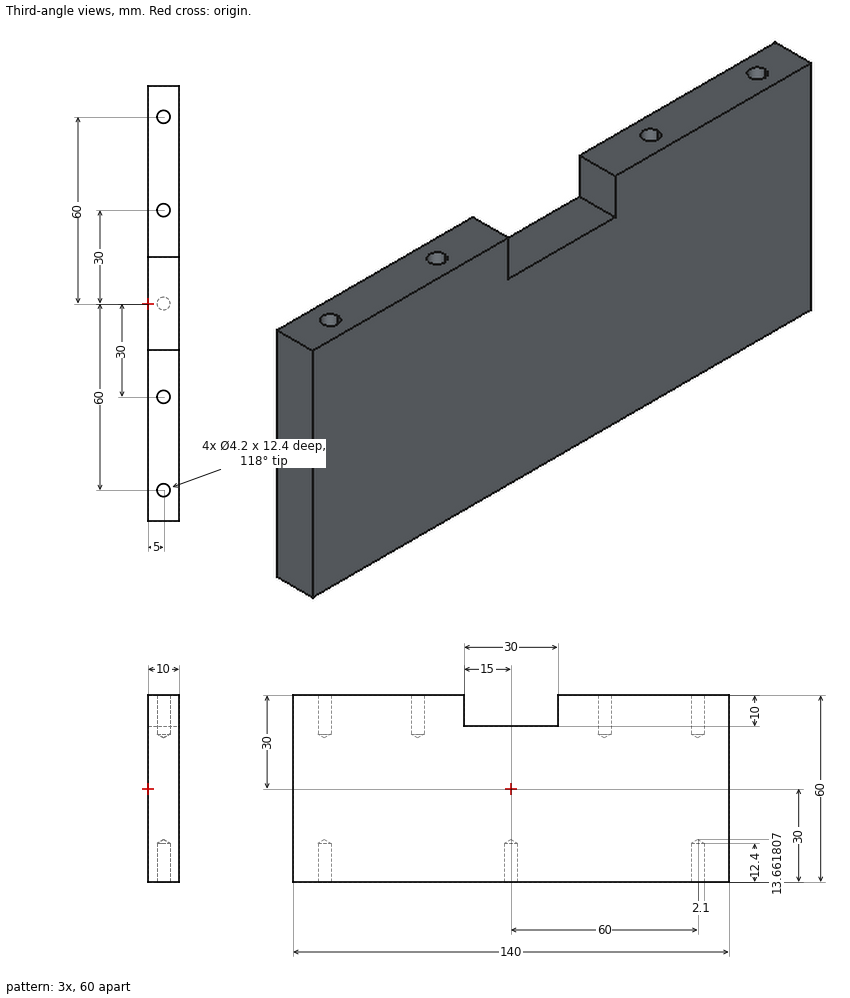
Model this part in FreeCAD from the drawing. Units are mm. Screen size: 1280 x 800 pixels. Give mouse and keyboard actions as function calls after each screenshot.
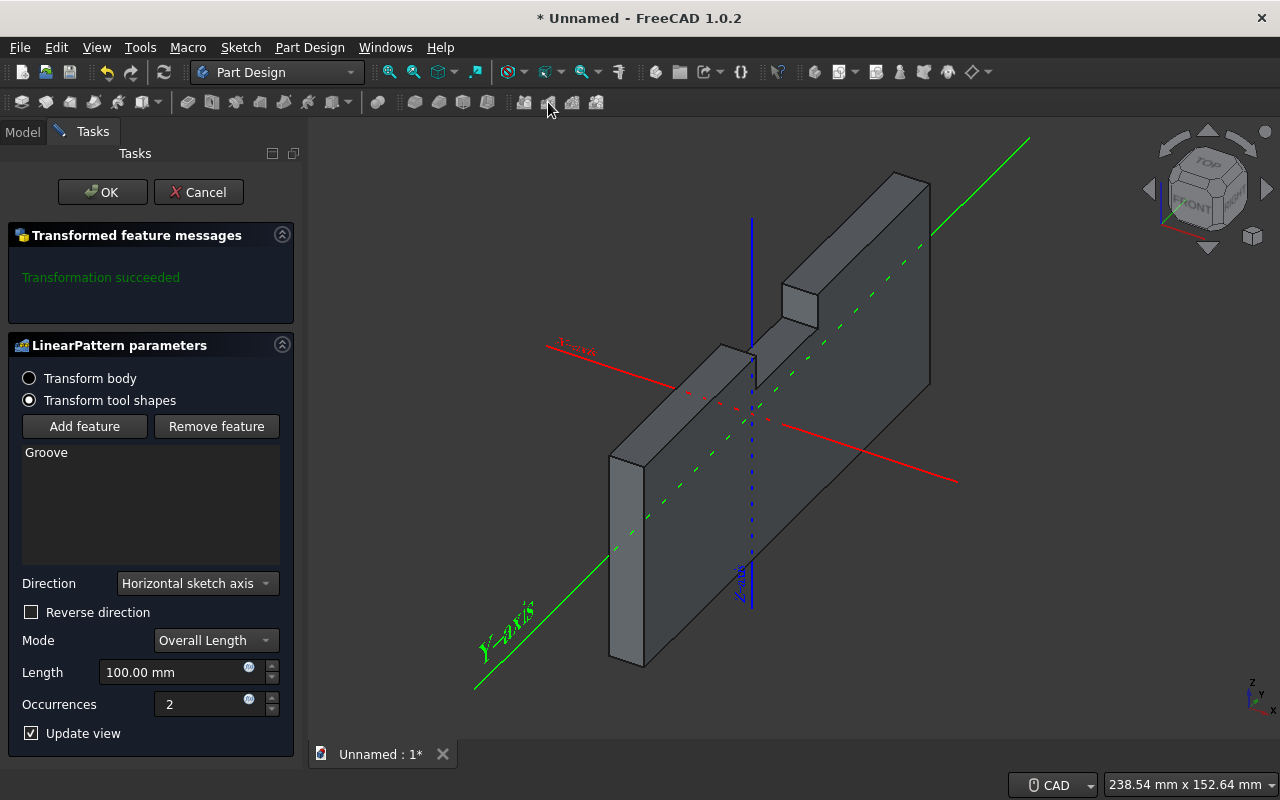
click(198, 584)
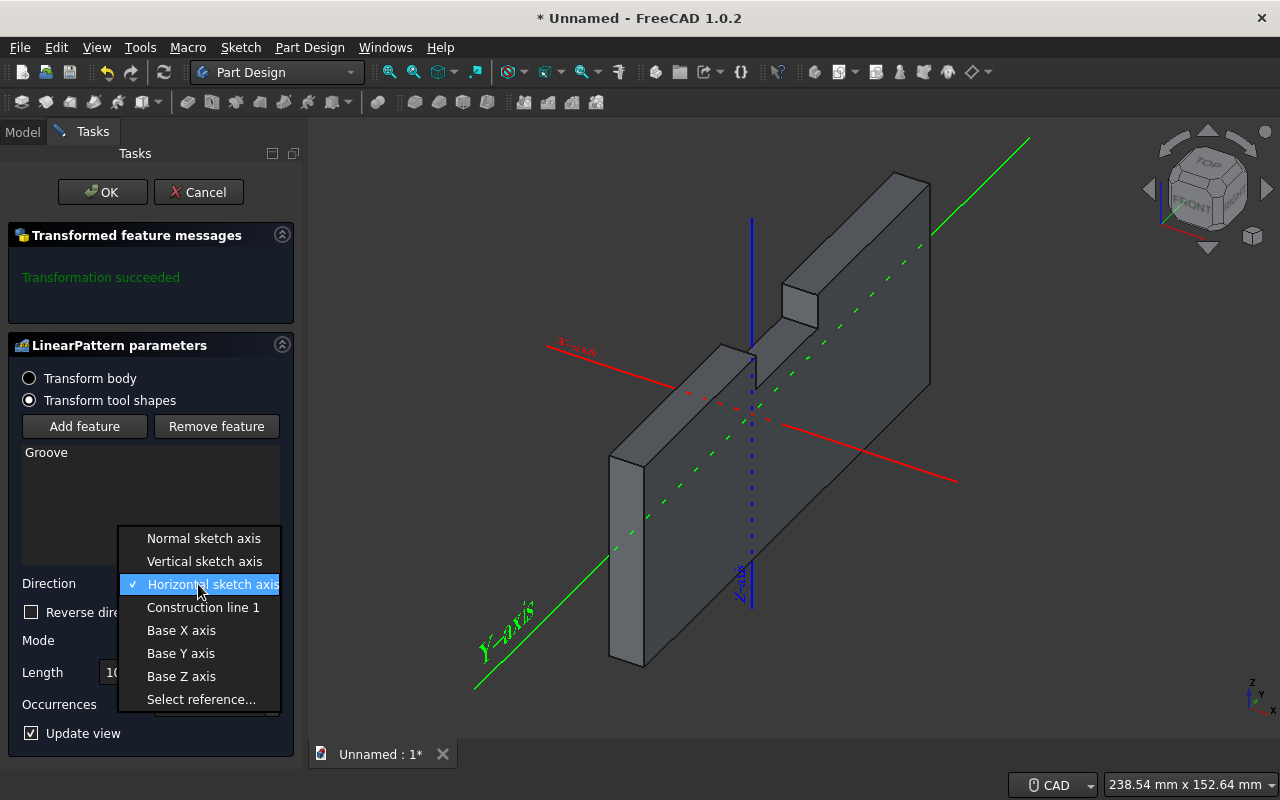
click(198, 654)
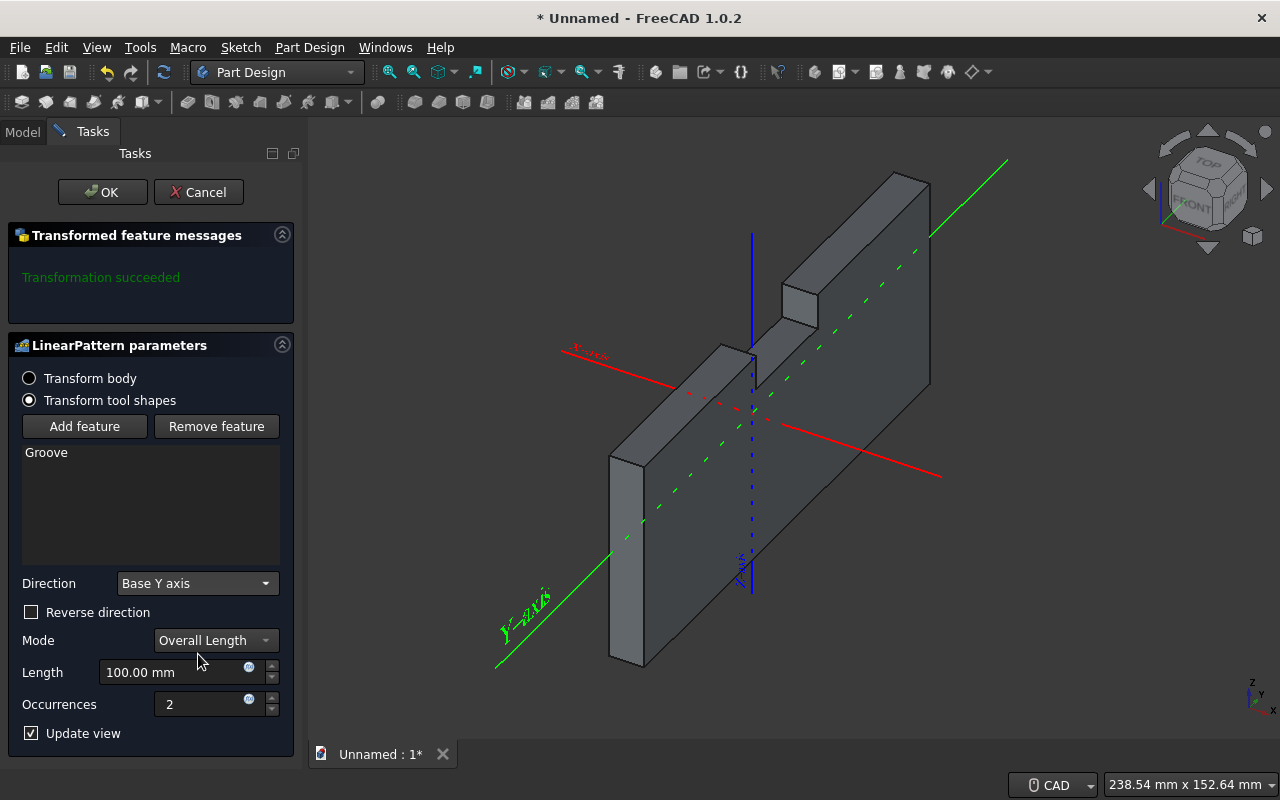
click(217, 640)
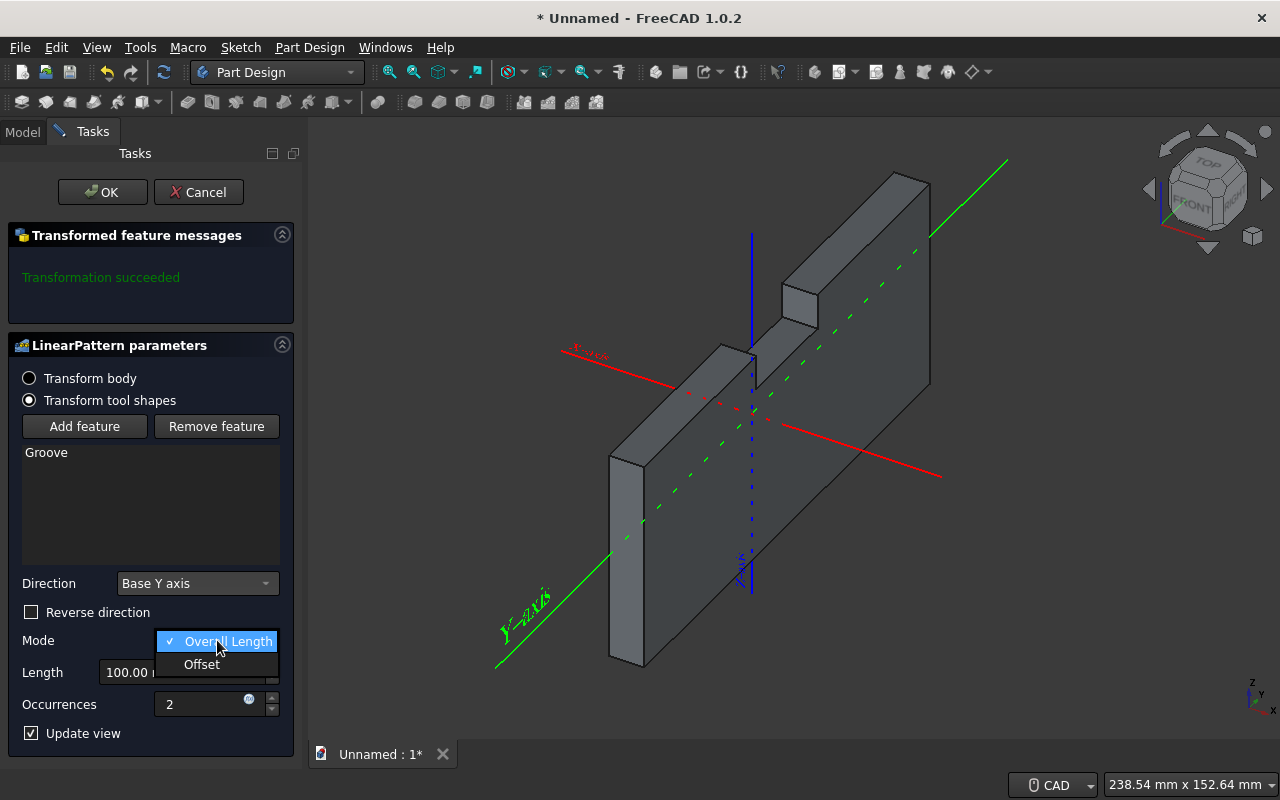
click(216, 664)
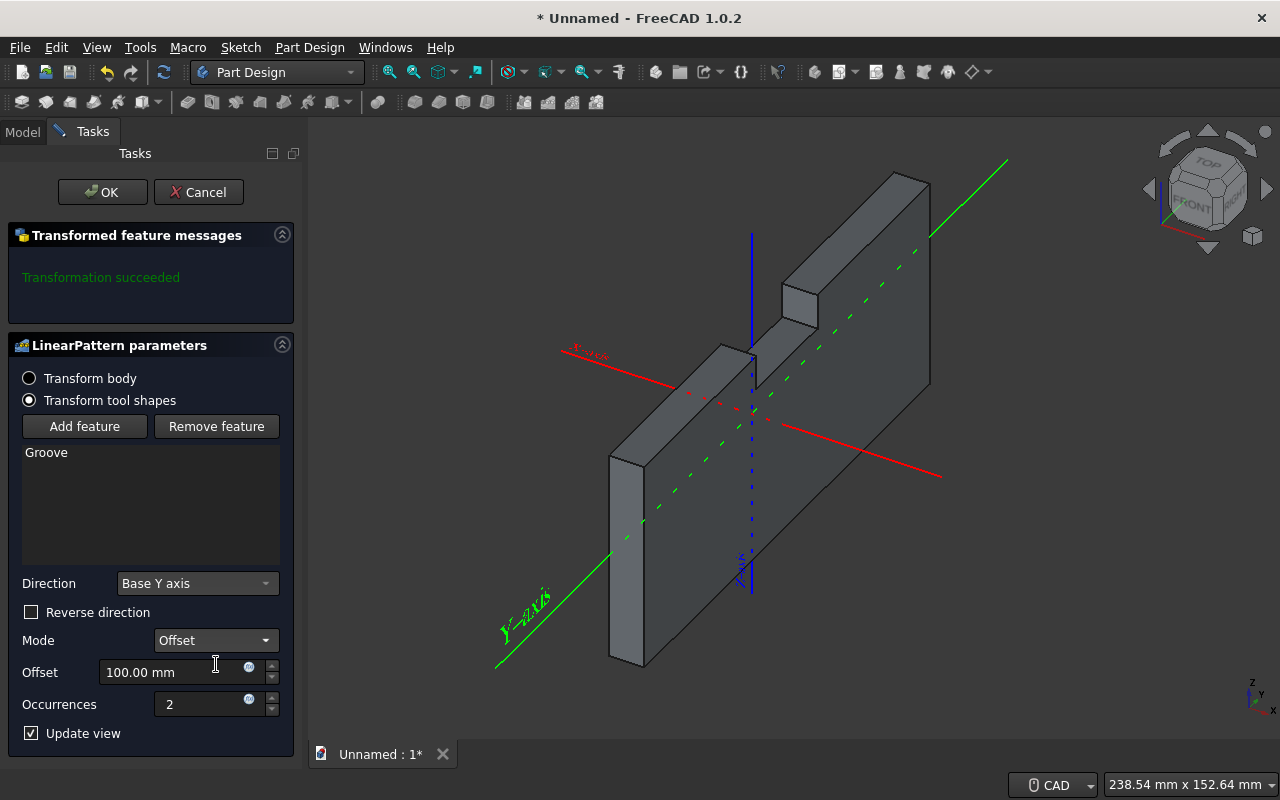
triple_click(182, 672)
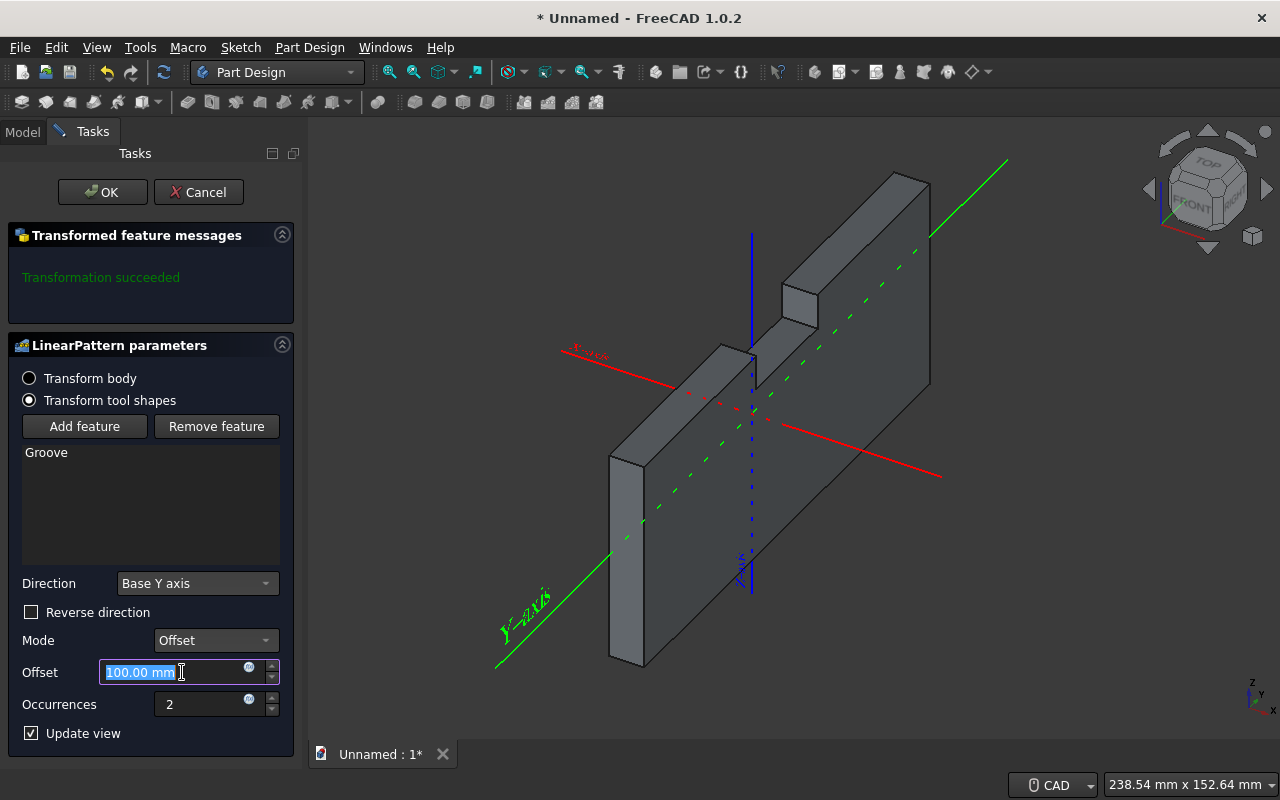
text(60)
key(Tab)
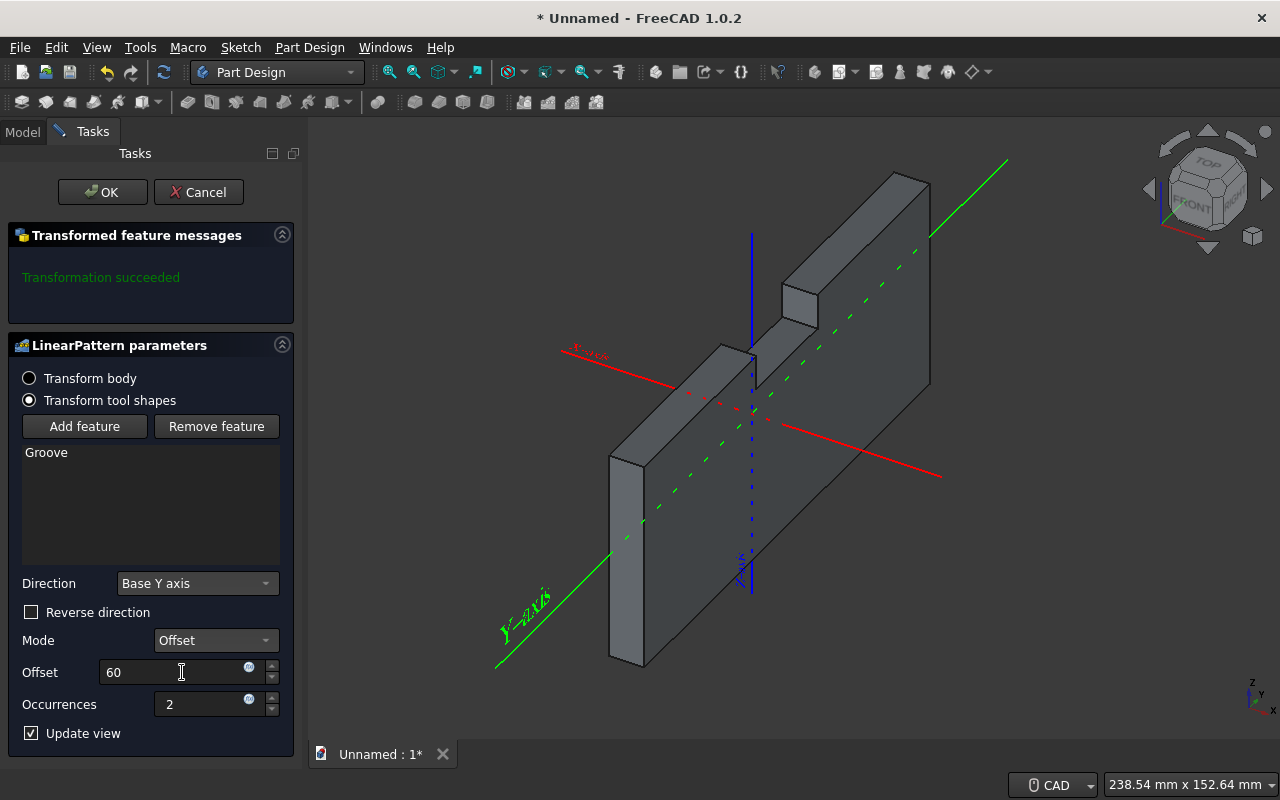
triple_click(209, 704)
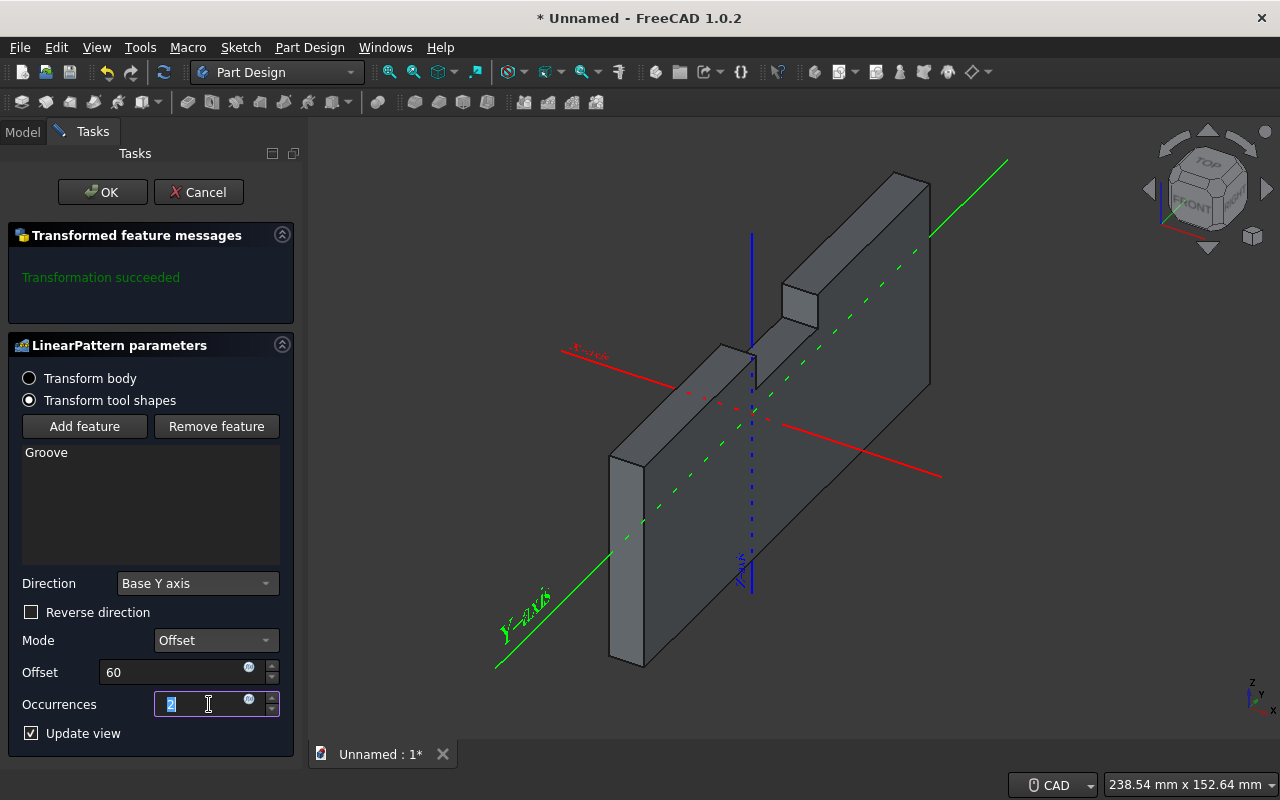
text(3)
key(Tab)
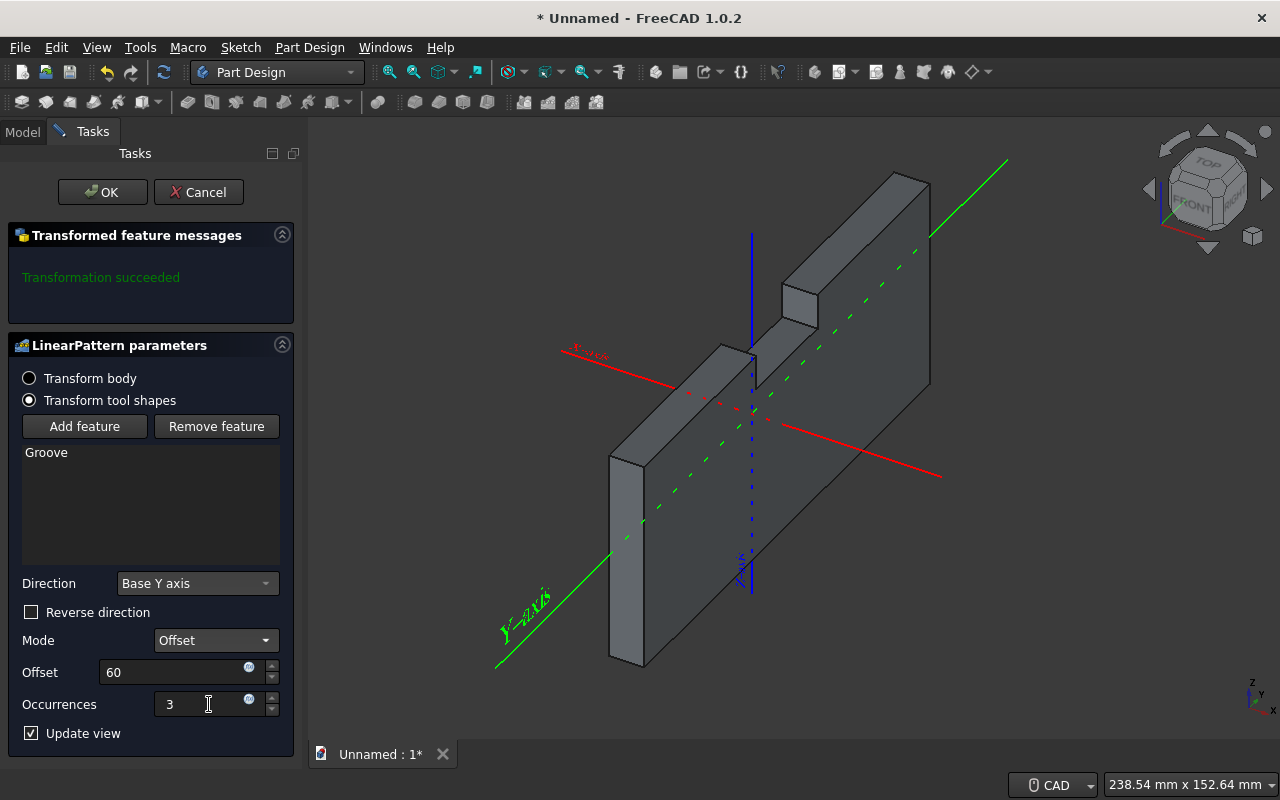
click(30, 612)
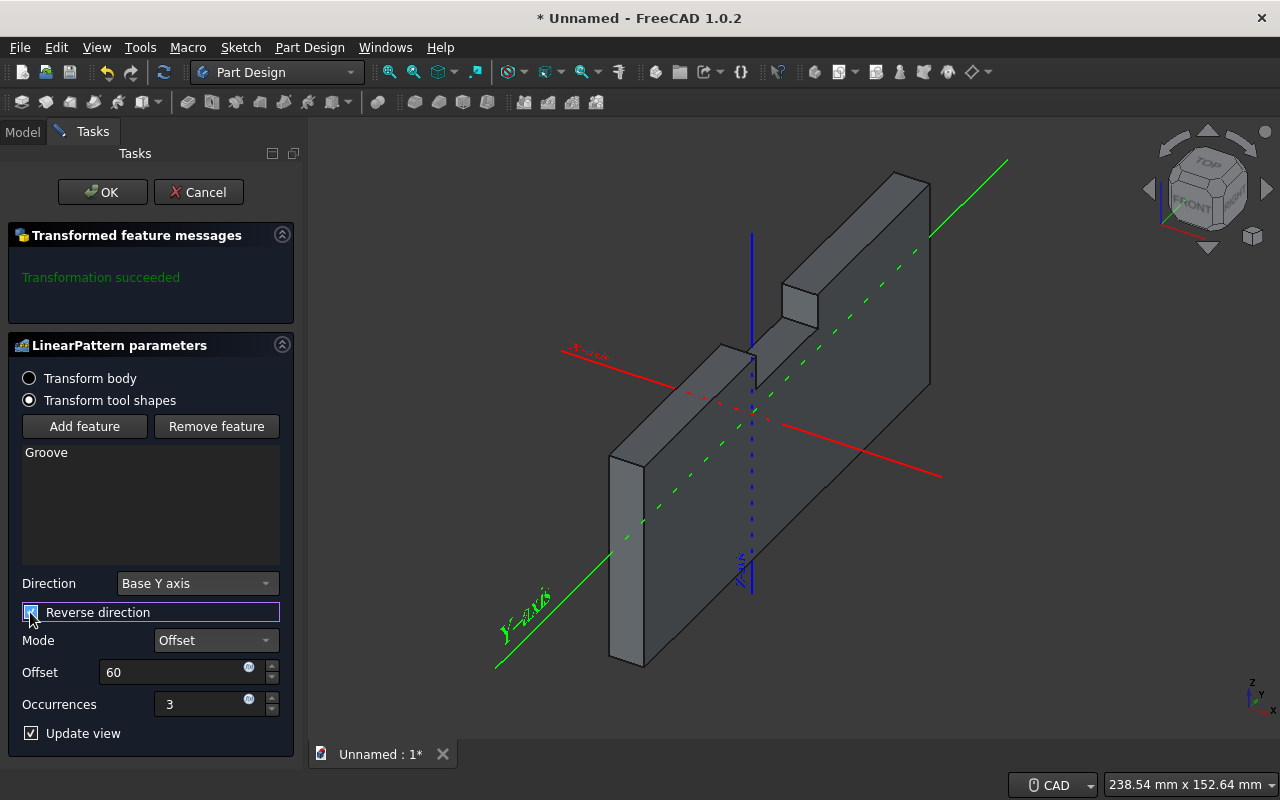
click(103, 192)